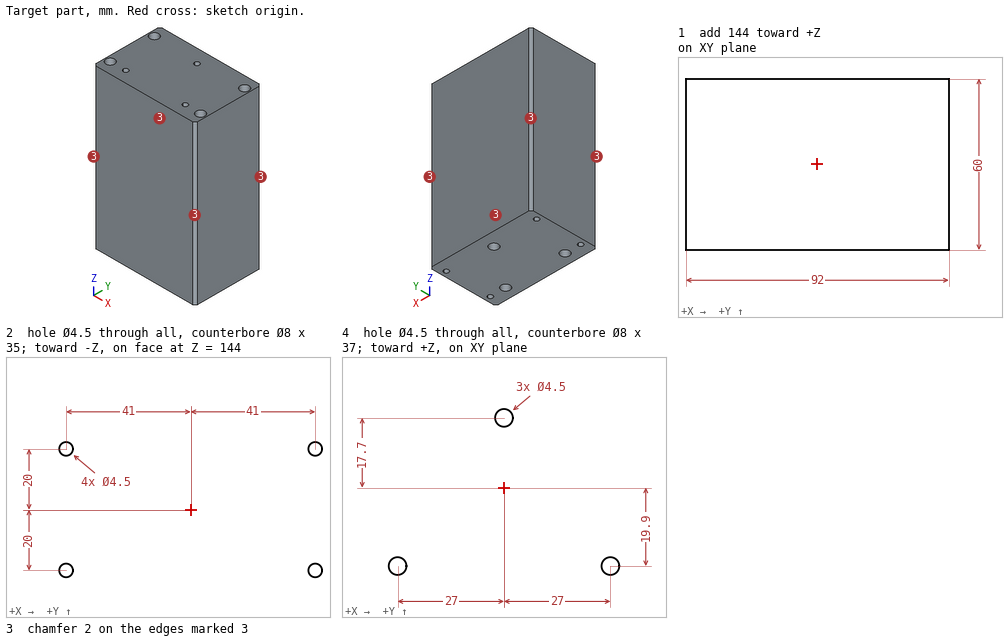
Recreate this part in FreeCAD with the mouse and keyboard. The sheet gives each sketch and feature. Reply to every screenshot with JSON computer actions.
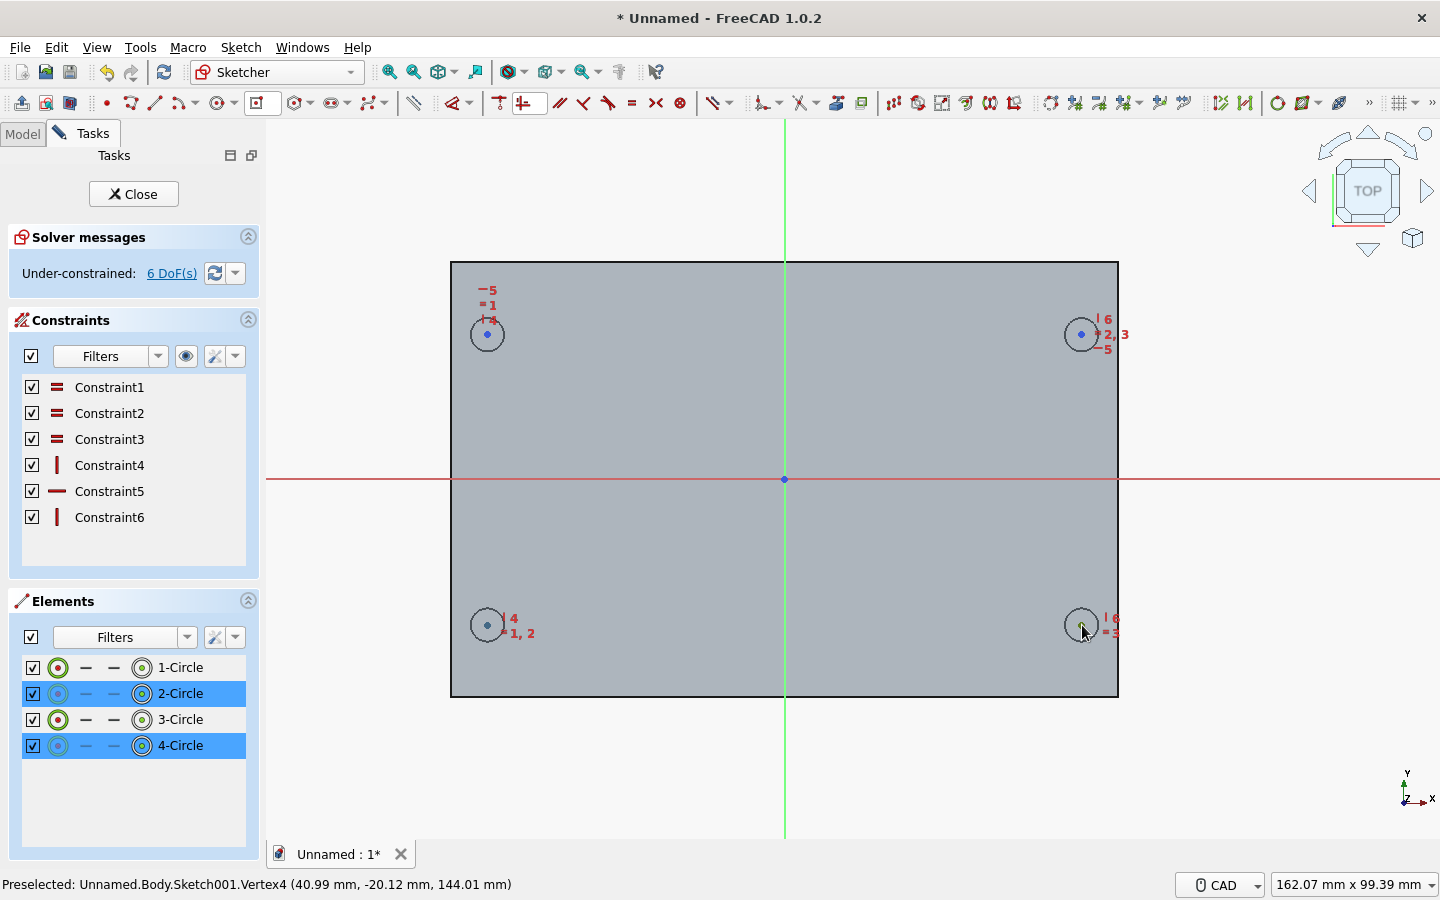
{"action": "key", "text": "h"}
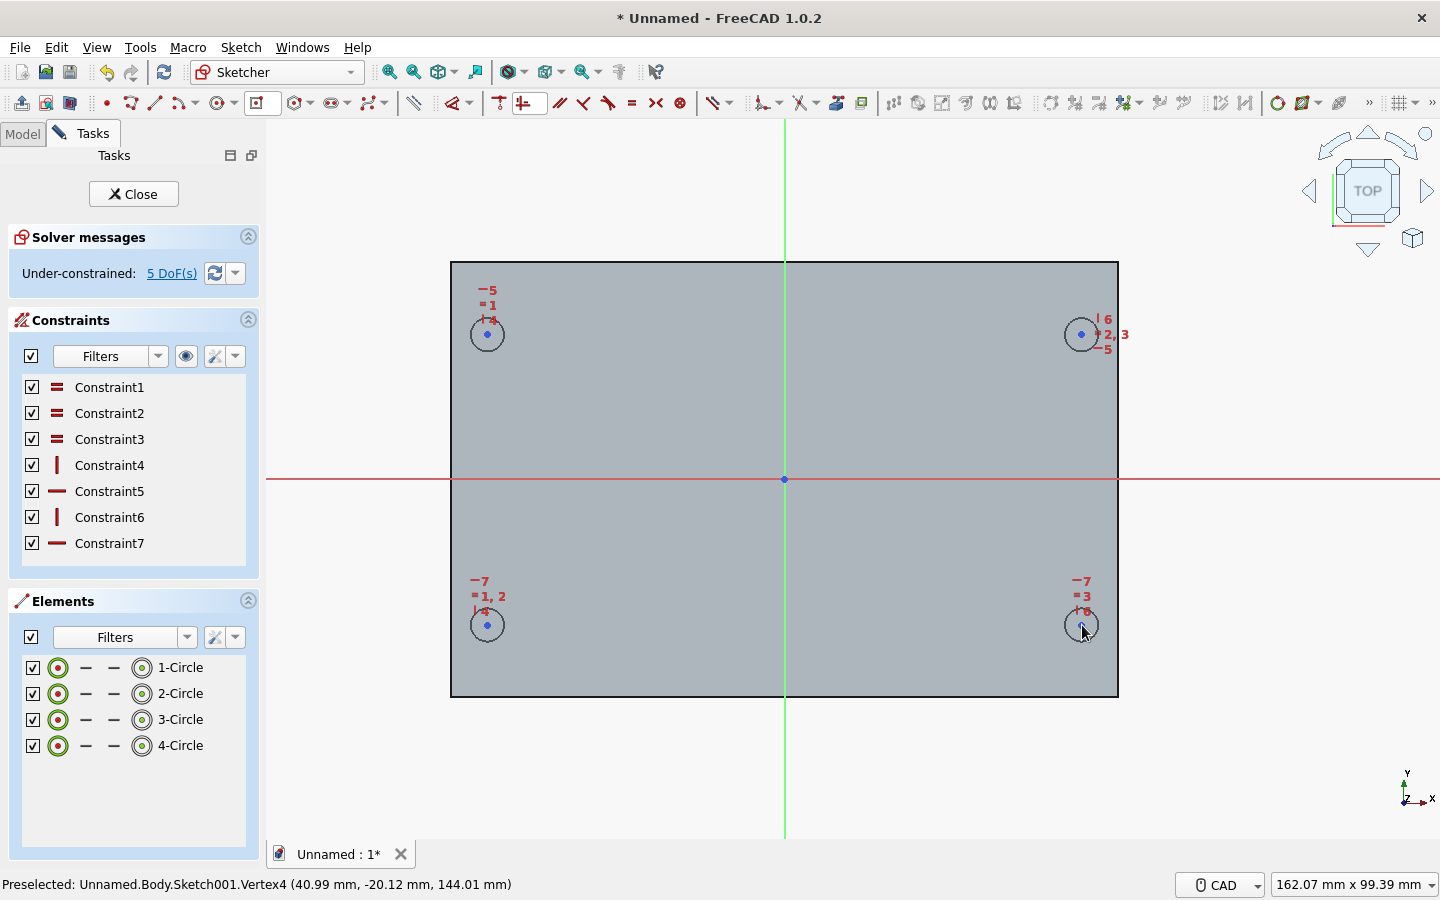
{"action": "left_click", "coordinate": [452, 104]}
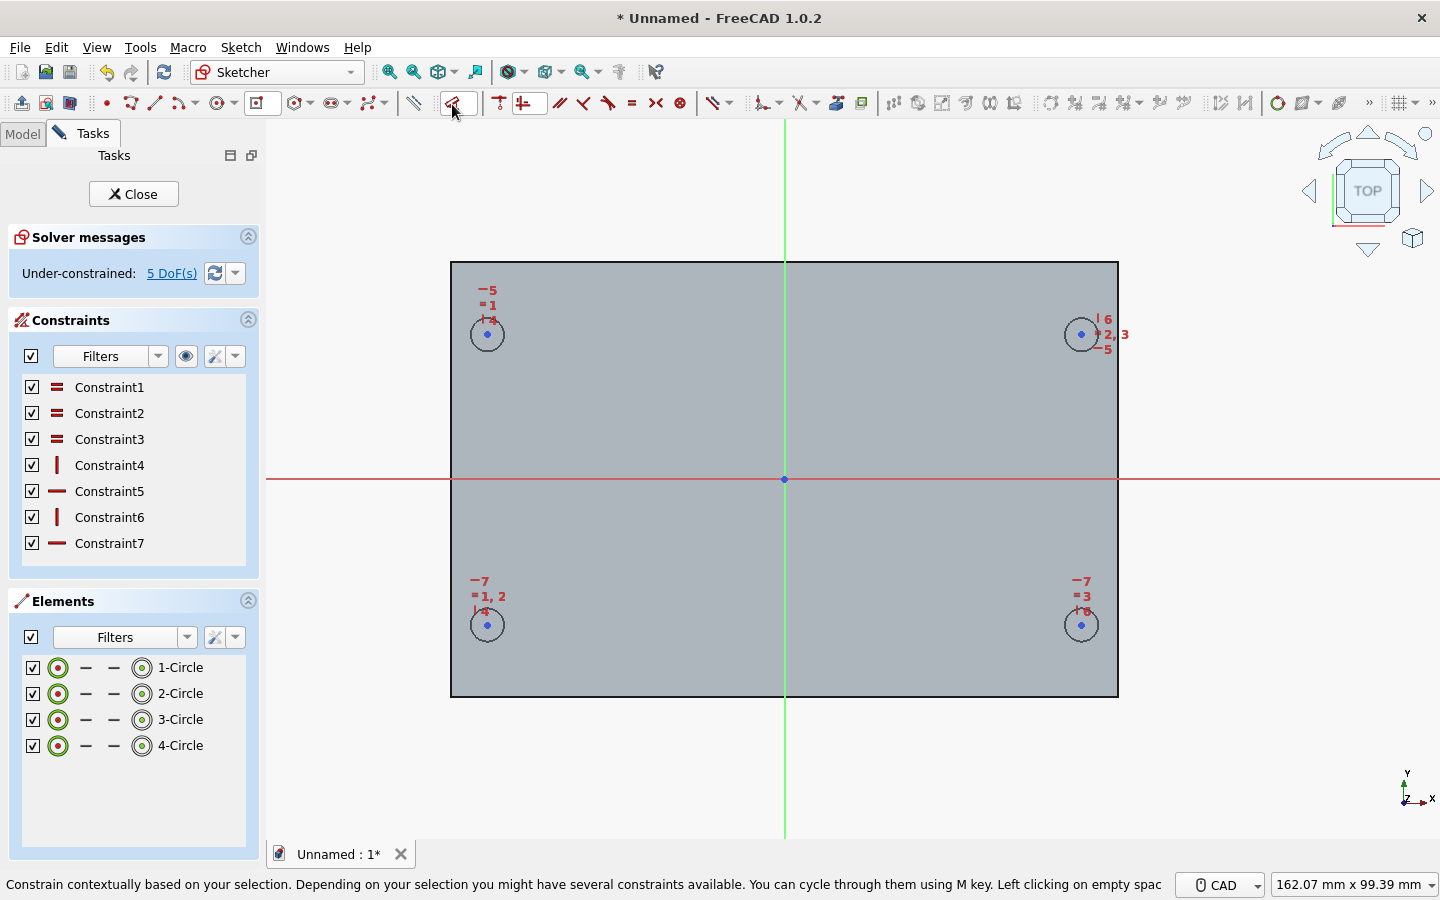
{"action": "left_click", "coordinate": [499, 323]}
{"action": "left_click", "coordinate": [521, 300]}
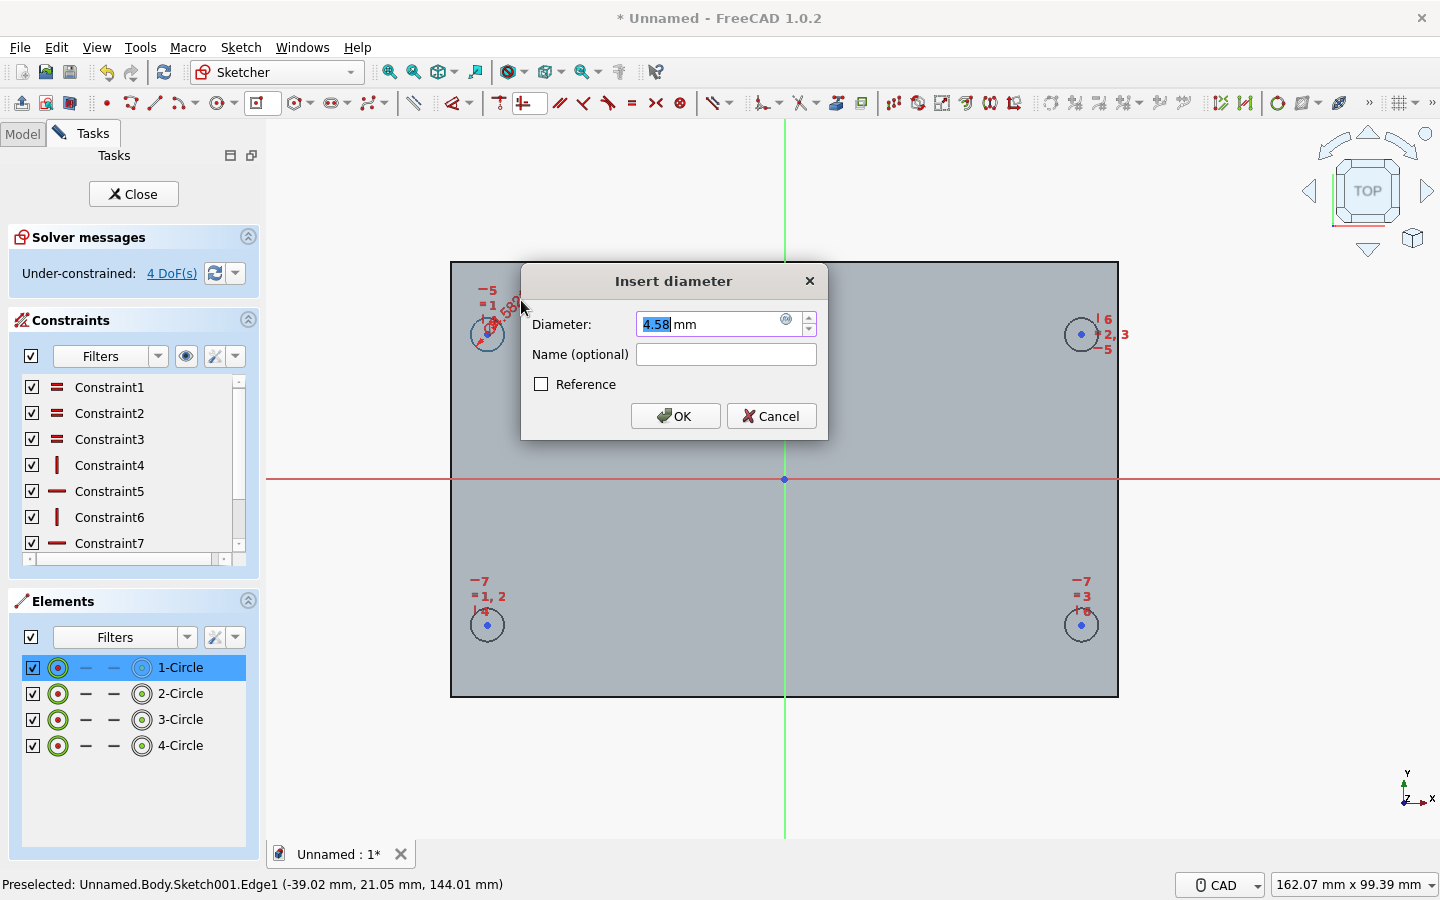
{"action": "type", "text": "4.5"}
{"action": "key", "text": "Return"}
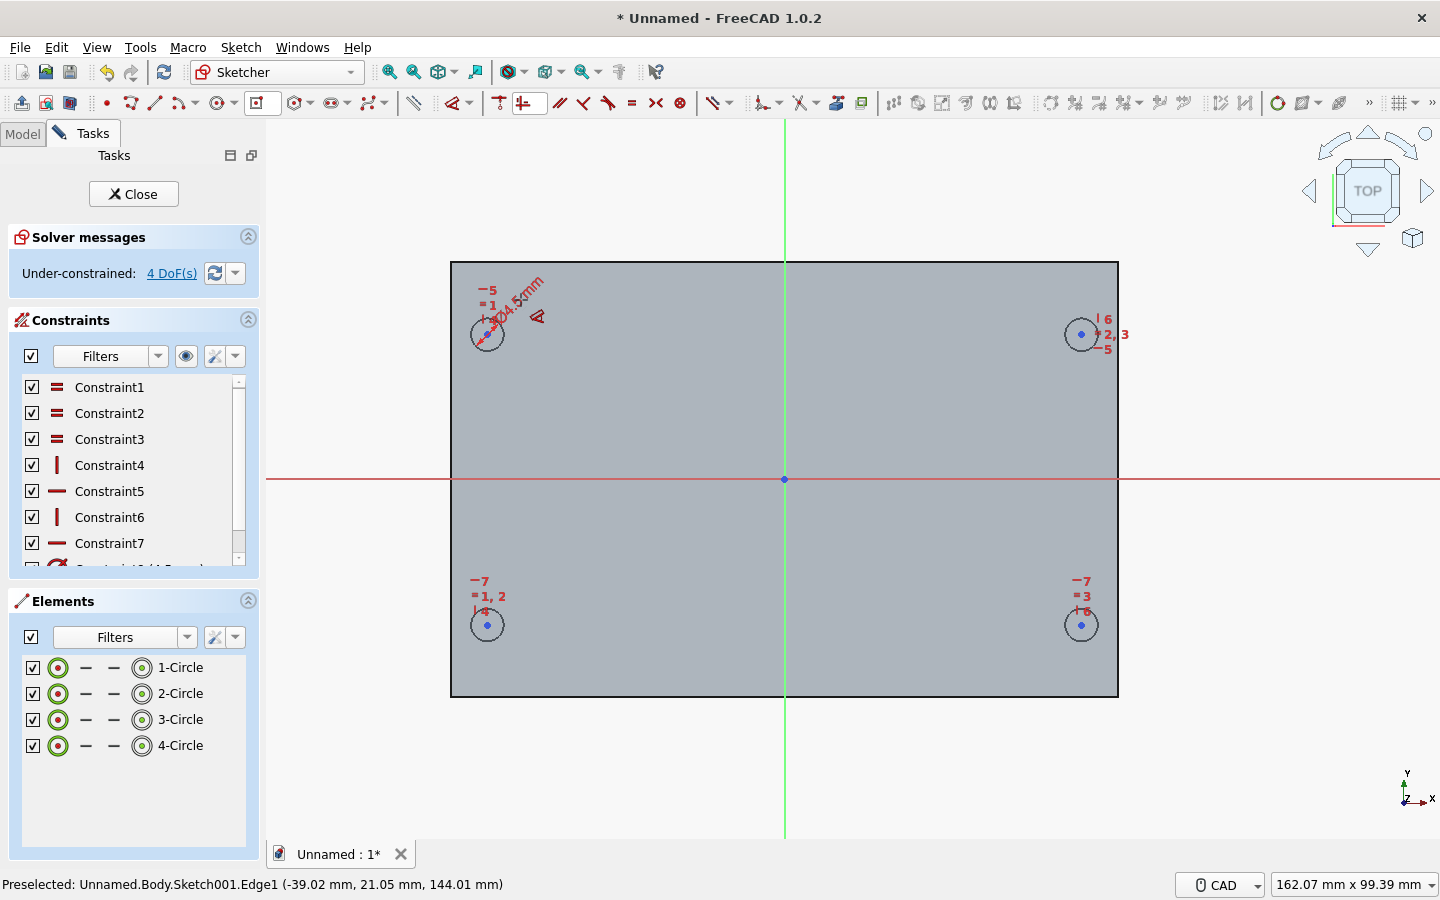
{"action": "left_click", "coordinate": [487, 335]}
{"action": "left_click", "coordinate": [636, 301]}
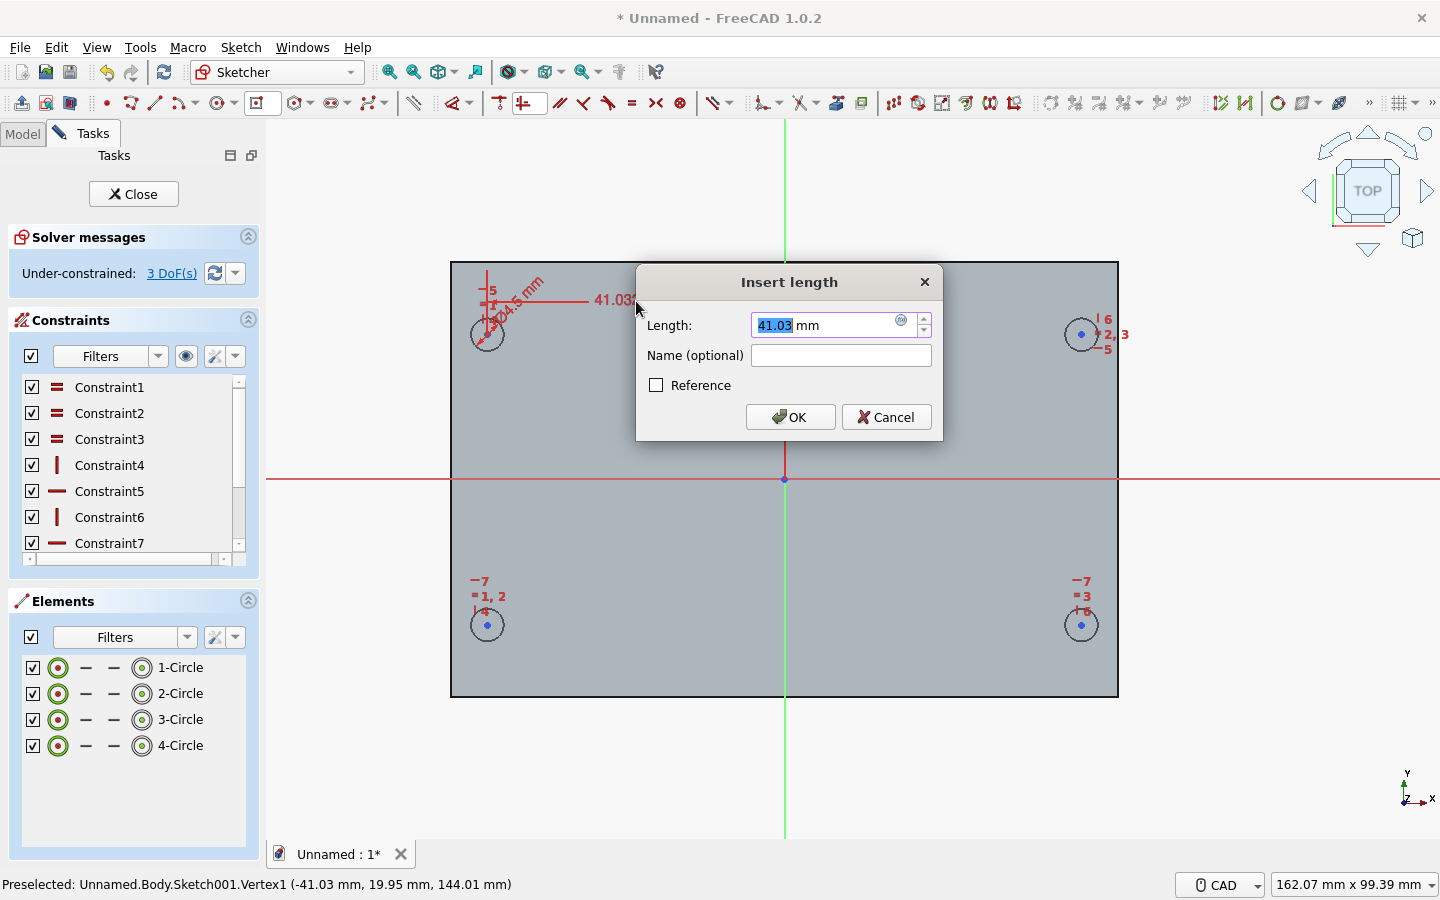
{"action": "type", "text": "41"}
{"action": "key", "text": "Return"}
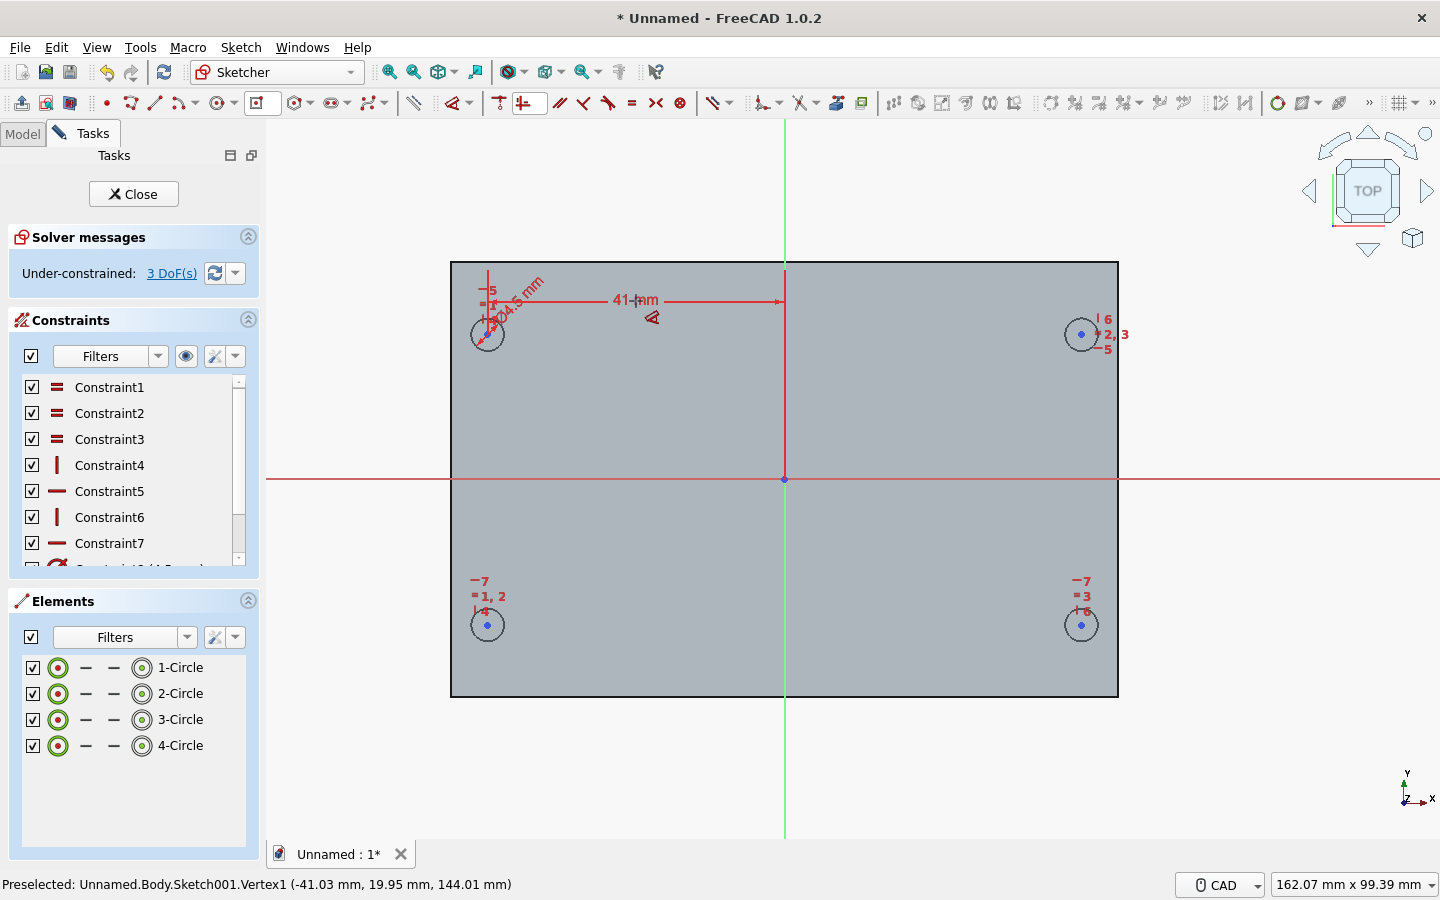
{"action": "left_click", "coordinate": [488, 335]}
{"action": "left_click", "coordinate": [454, 407]}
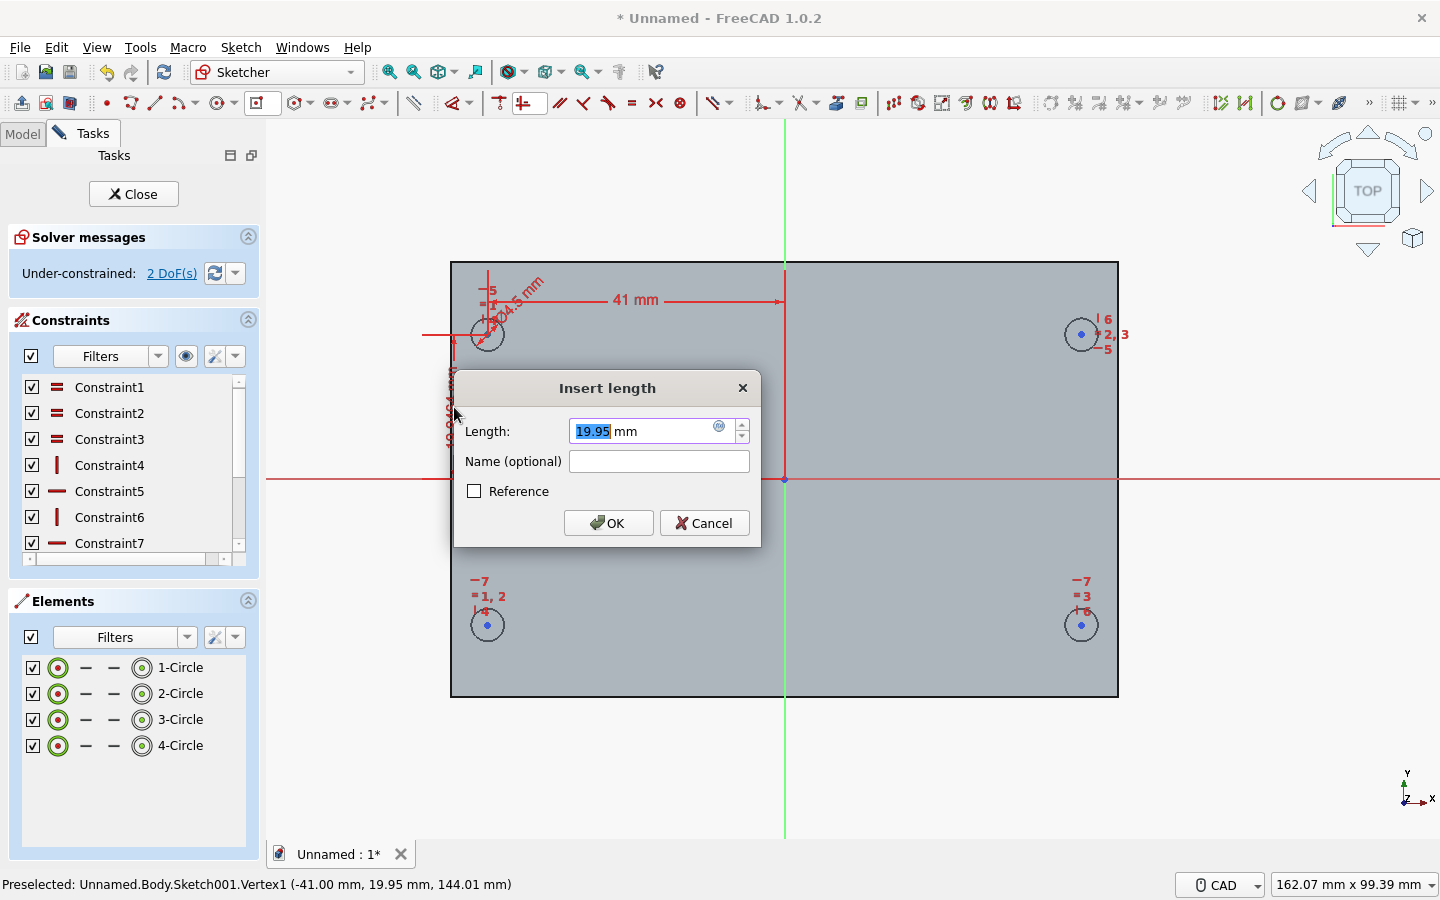
{"action": "type", "text": "20"}
{"action": "key", "text": "Return"}